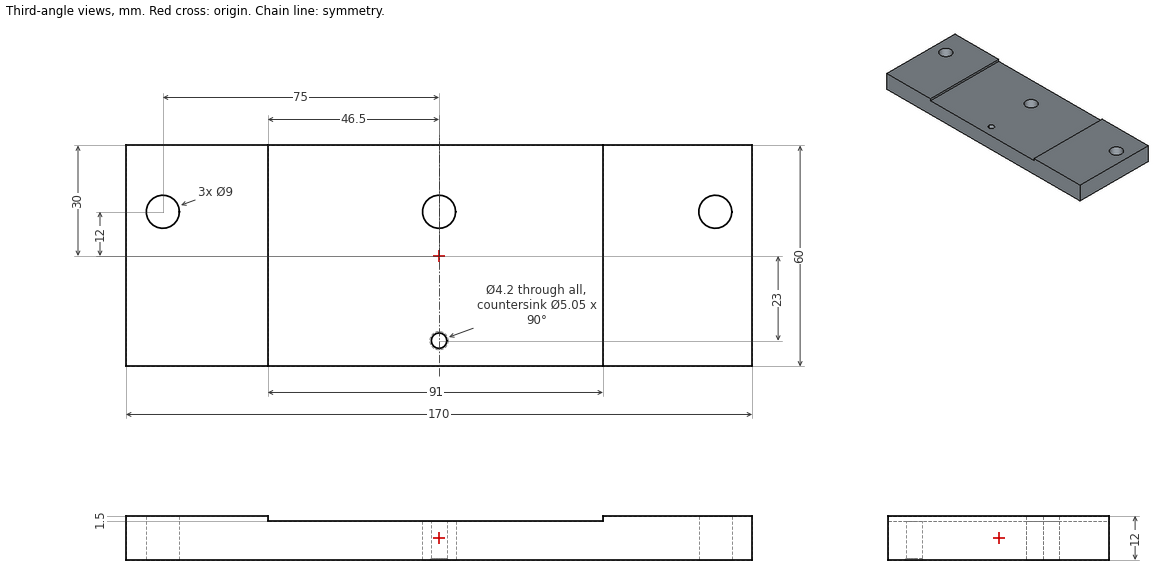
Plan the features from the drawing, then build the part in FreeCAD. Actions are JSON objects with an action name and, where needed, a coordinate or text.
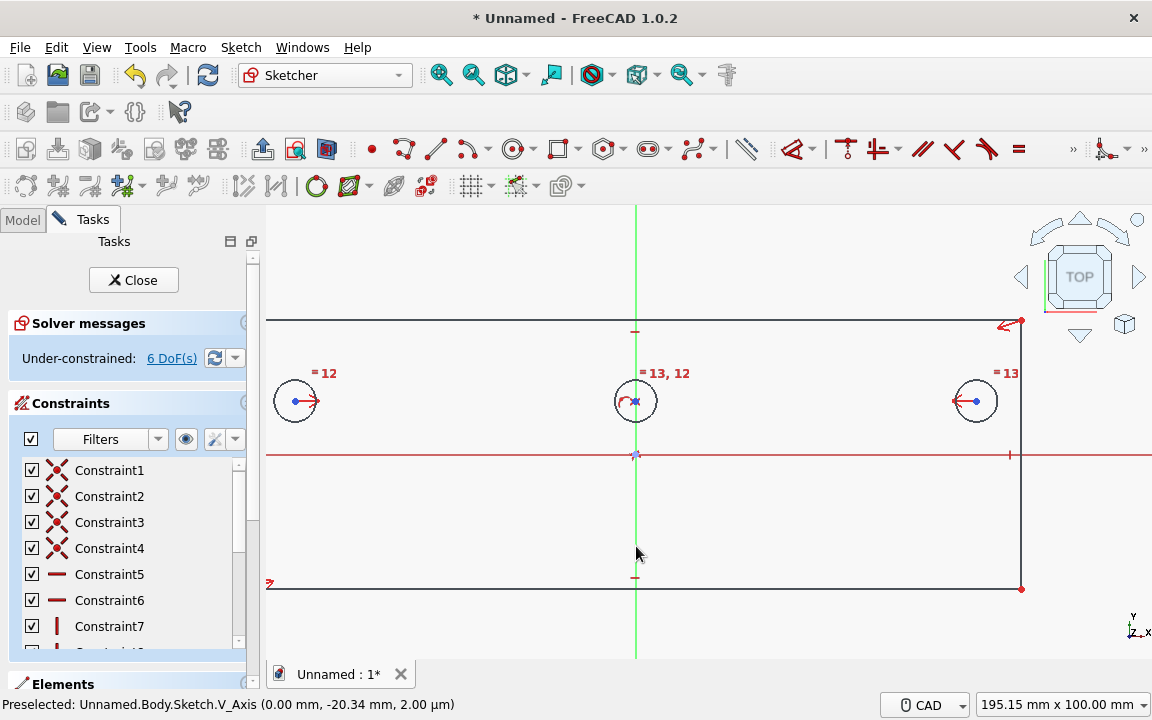
{"action": "left_click", "coordinate": [792, 150]}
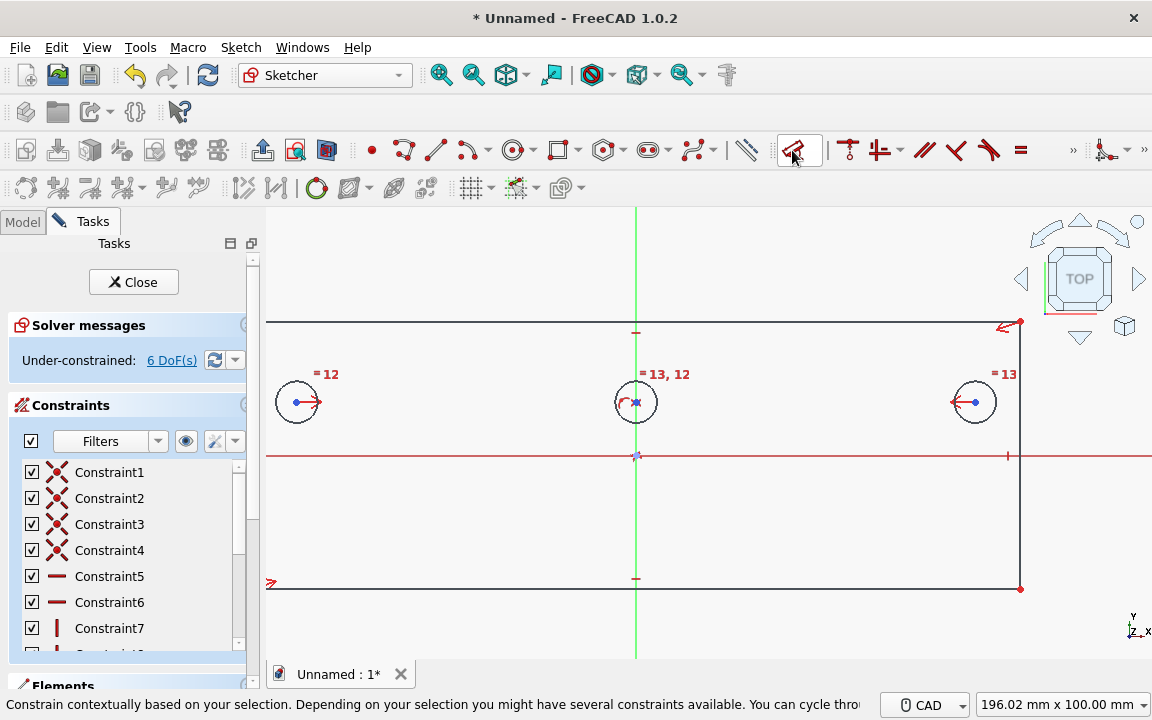
{"action": "left_click", "coordinate": [311, 387]}
{"action": "left_click", "coordinate": [333, 364]}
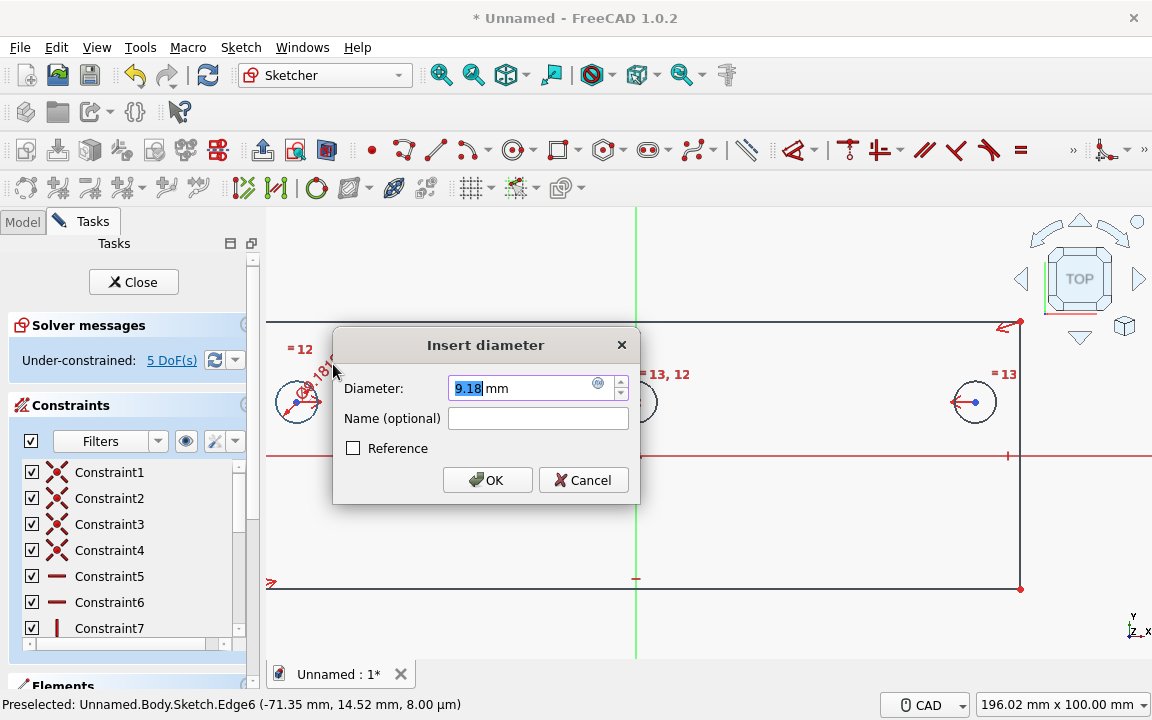
{"action": "type", "text": "9"}
{"action": "key", "text": "Return"}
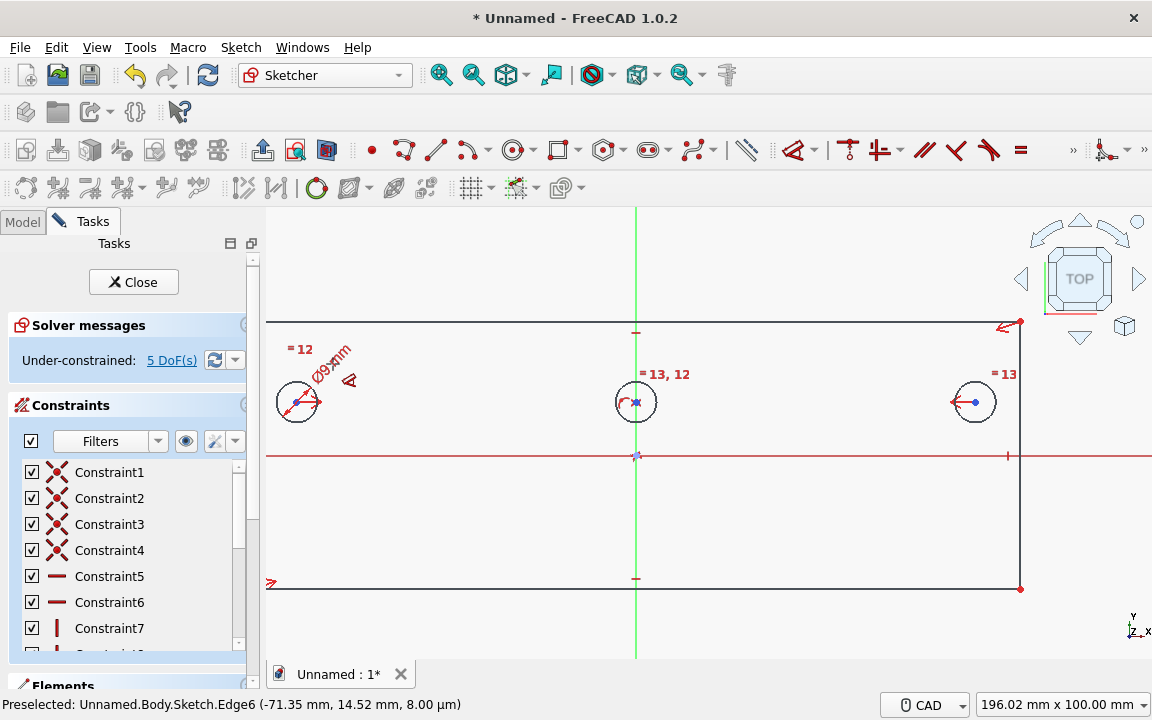
{"action": "scroll", "coordinate": [649, 387], "scroll_direction": "down", "scroll_amount": 2}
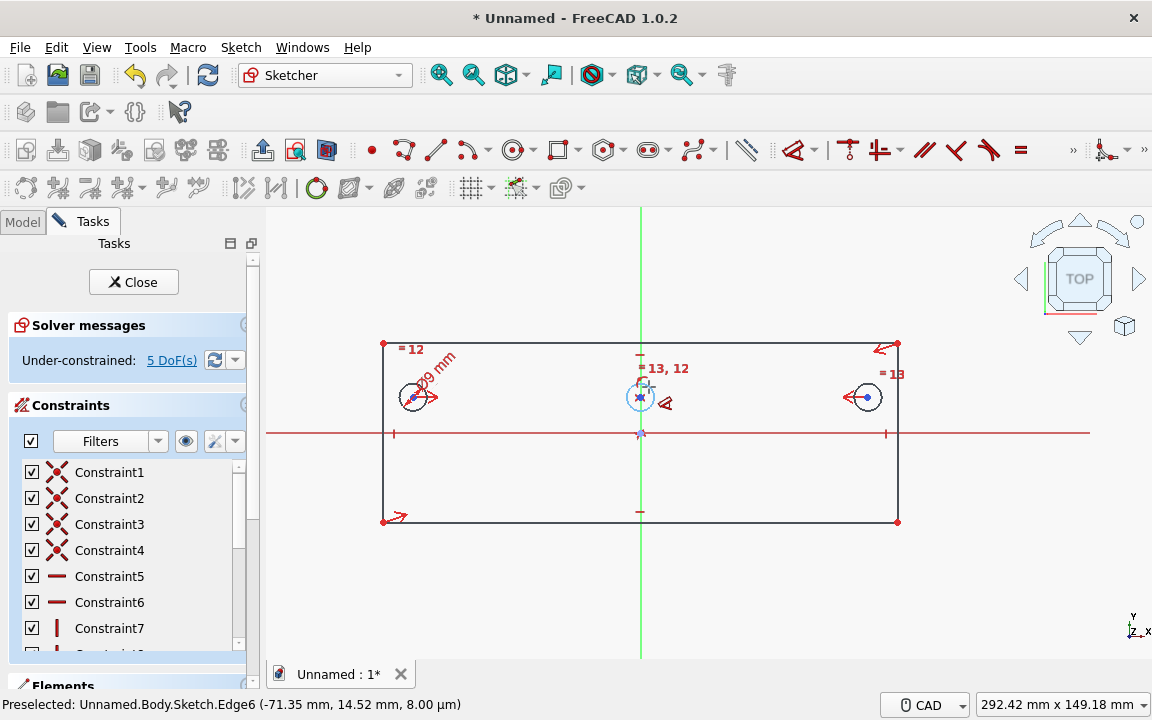
{"action": "left_click", "coordinate": [898, 469]}
{"action": "left_click", "coordinate": [932, 392]}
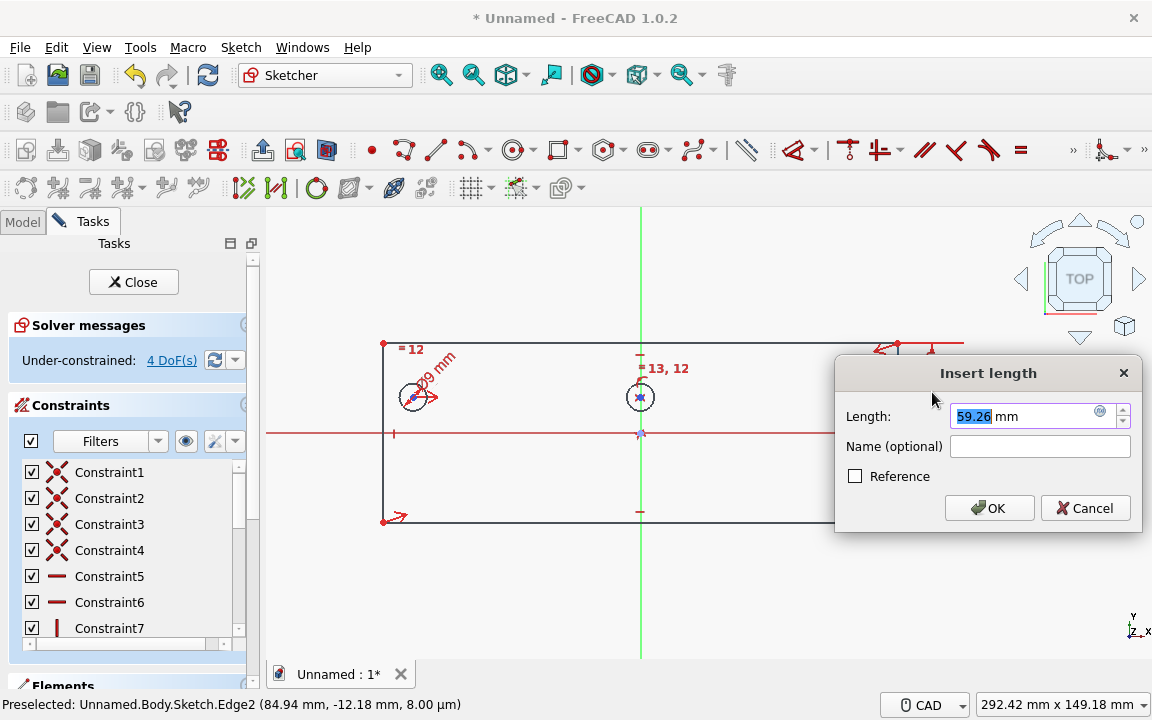
{"action": "type", "text": "60"}
{"action": "key", "text": "Return"}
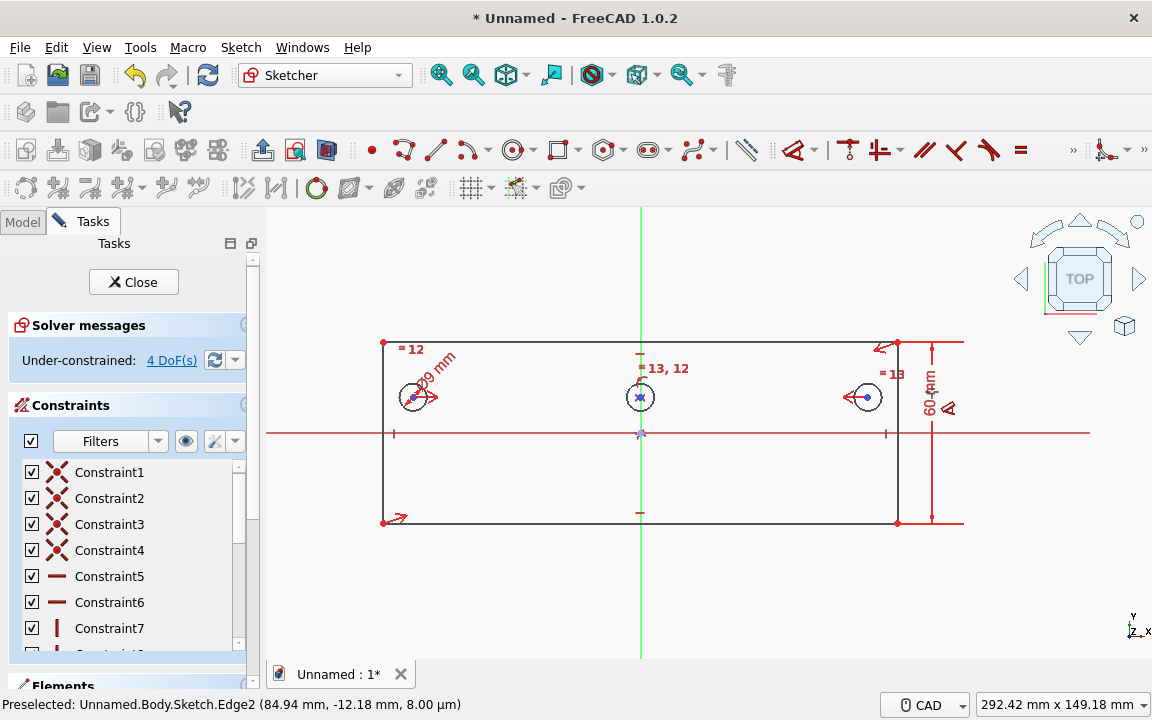
{"action": "left_click", "coordinate": [413, 397]}
{"action": "left_click", "coordinate": [527, 363]}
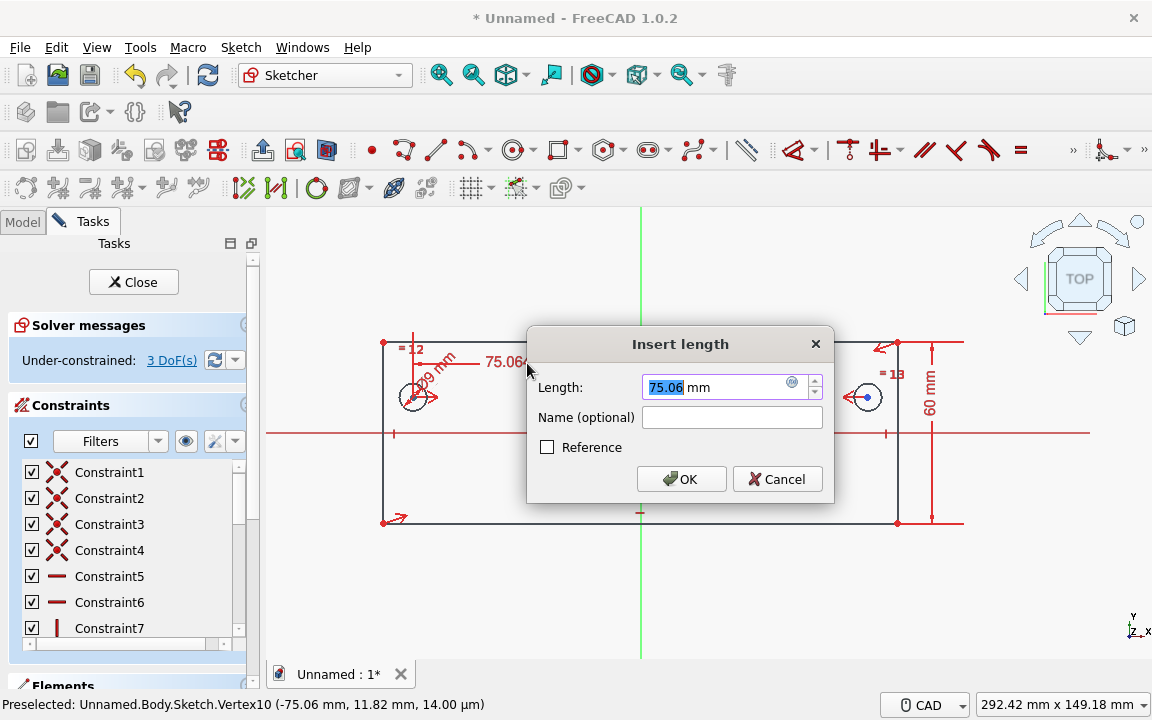
{"action": "type", "text": "75"}
{"action": "key", "text": "Return"}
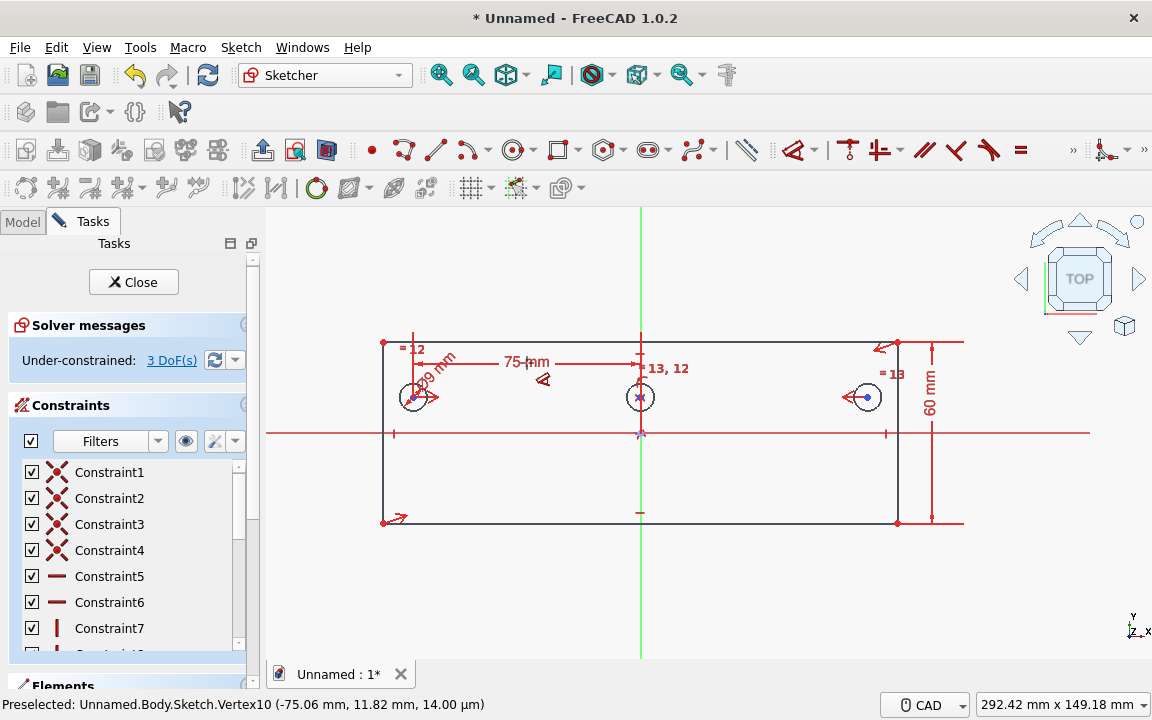
{"action": "left_click", "coordinate": [413, 397]}
{"action": "left_click", "coordinate": [675, 415]}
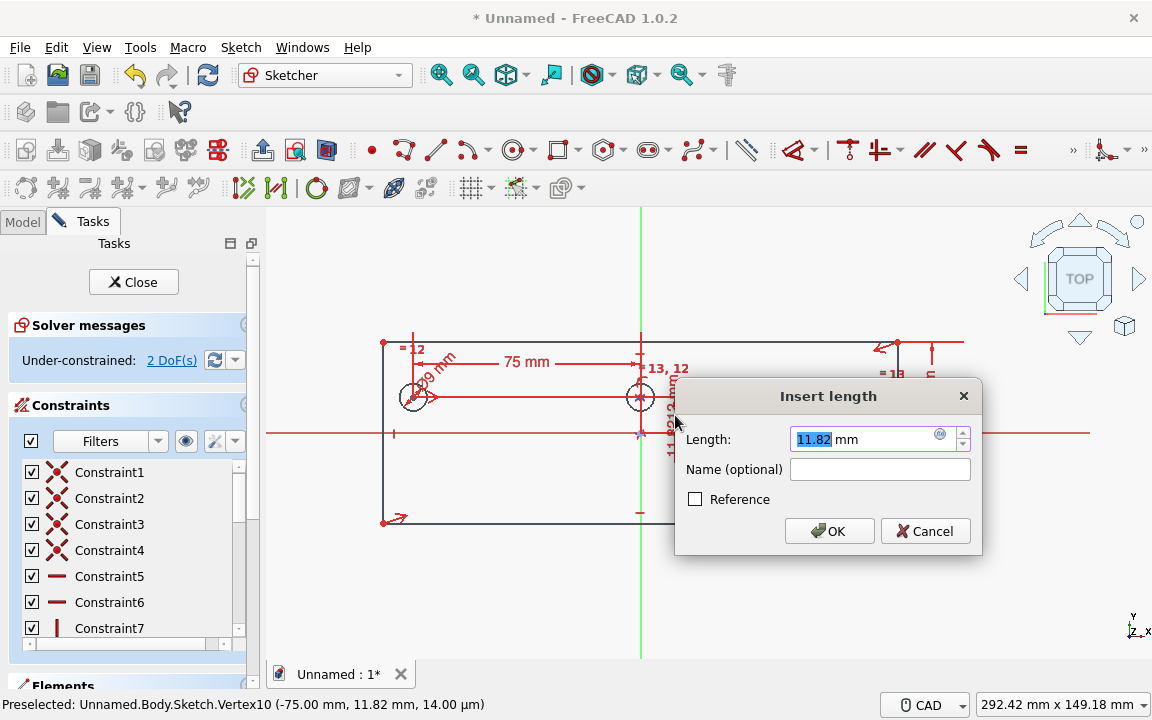
{"action": "type", "text": "12"}
{"action": "key", "text": "Return"}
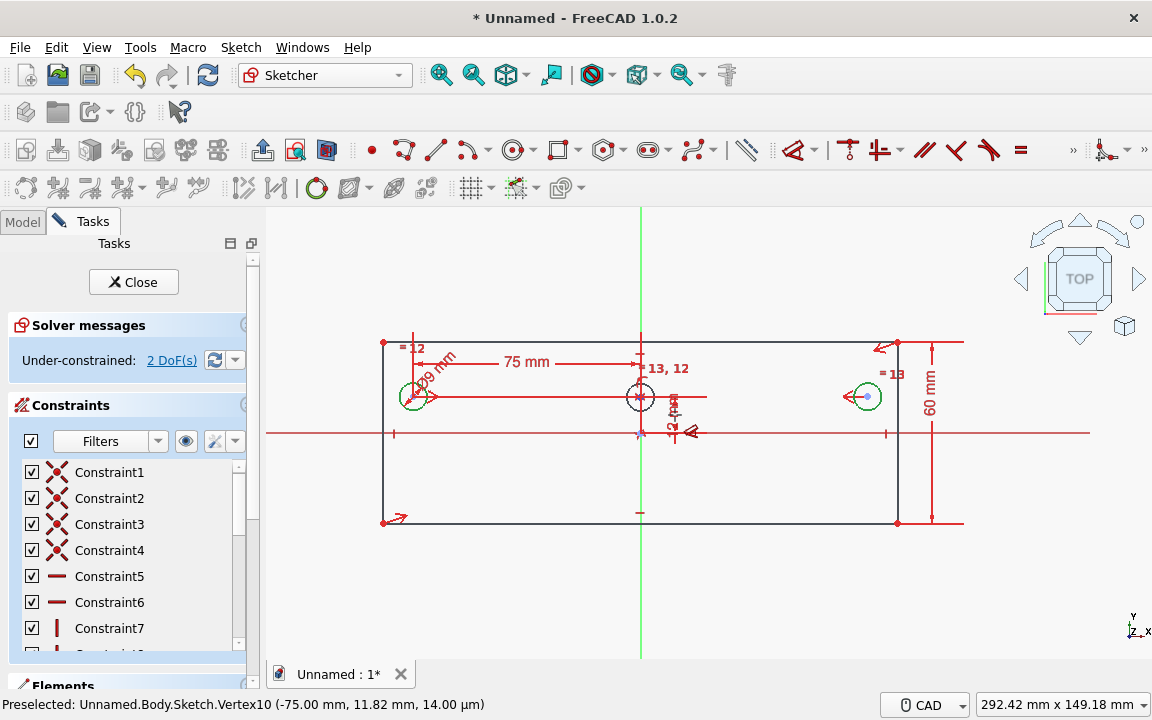
{"action": "left_click", "coordinate": [641, 397]}
{"action": "left_click", "coordinate": [583, 415]}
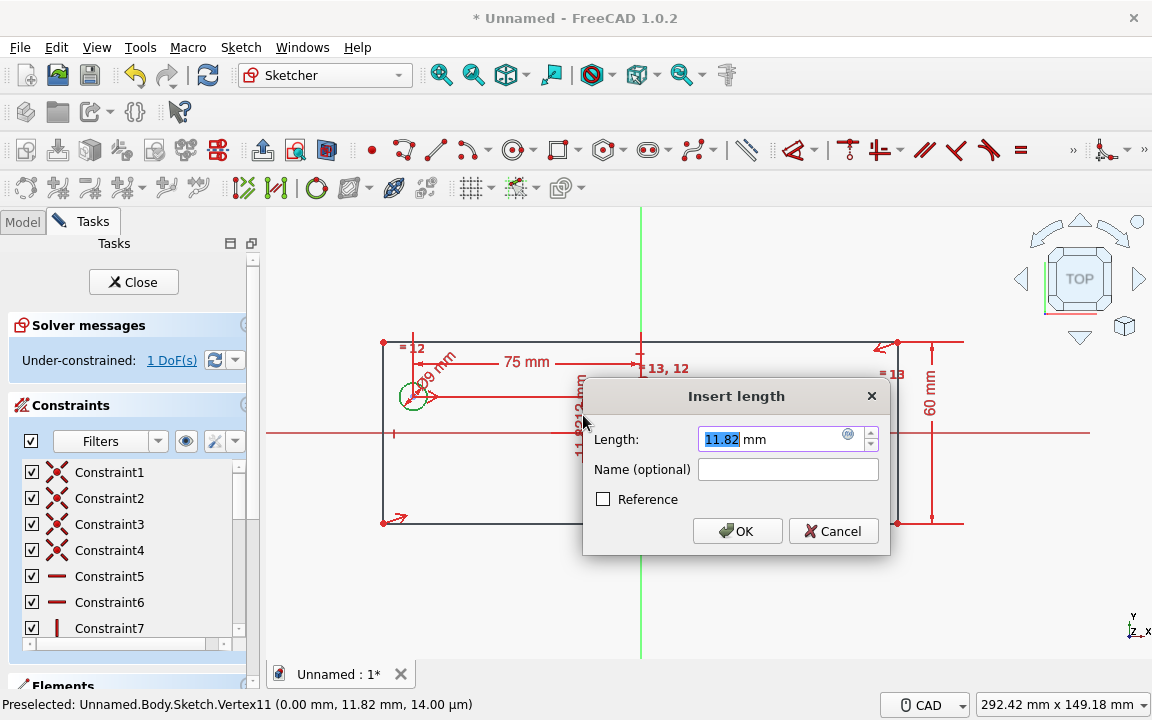
{"action": "type", "text": "12"}
{"action": "key", "text": "Return"}